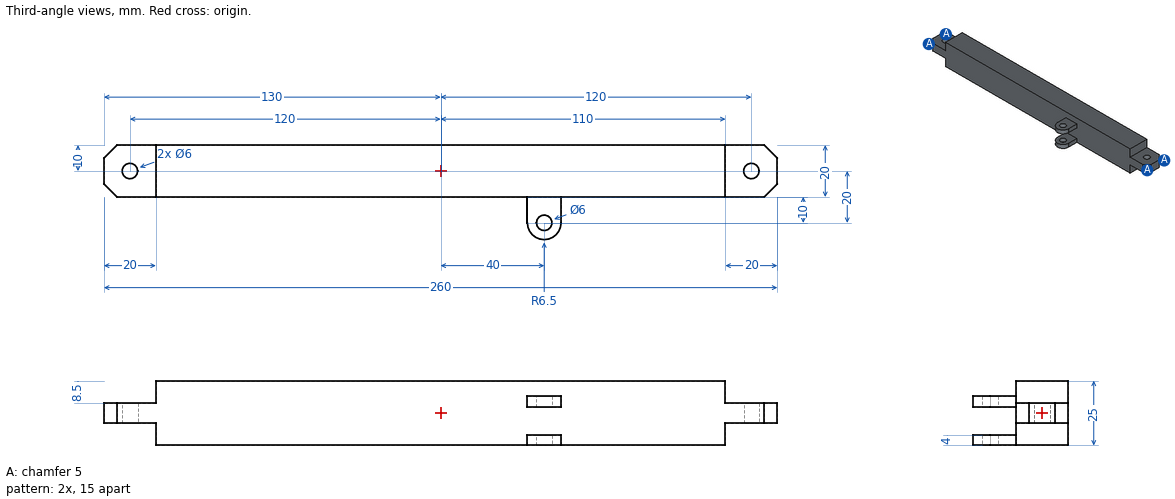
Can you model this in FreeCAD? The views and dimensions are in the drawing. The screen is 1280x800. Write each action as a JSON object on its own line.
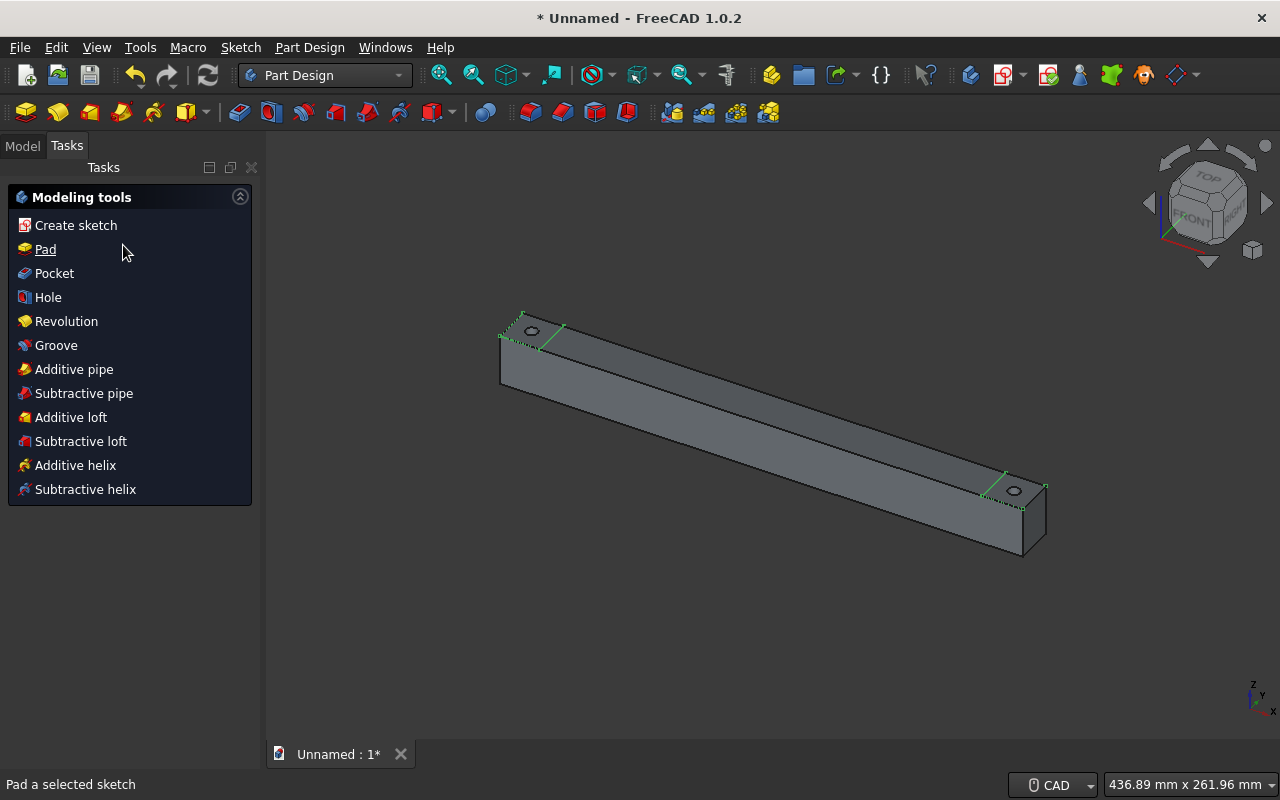
{"action": "left_click", "coordinate": [240, 112]}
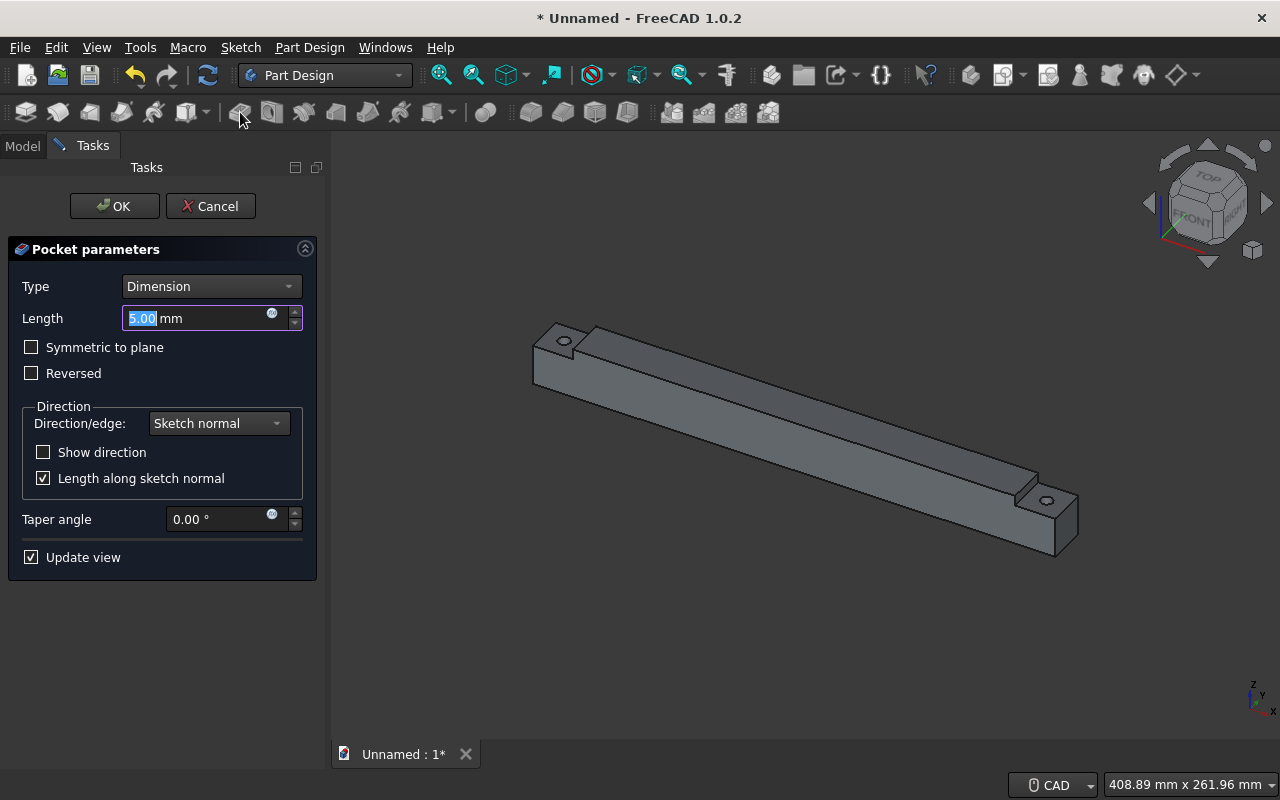
{"action": "type", "text": "8.5"}
{"action": "key", "text": "Tab"}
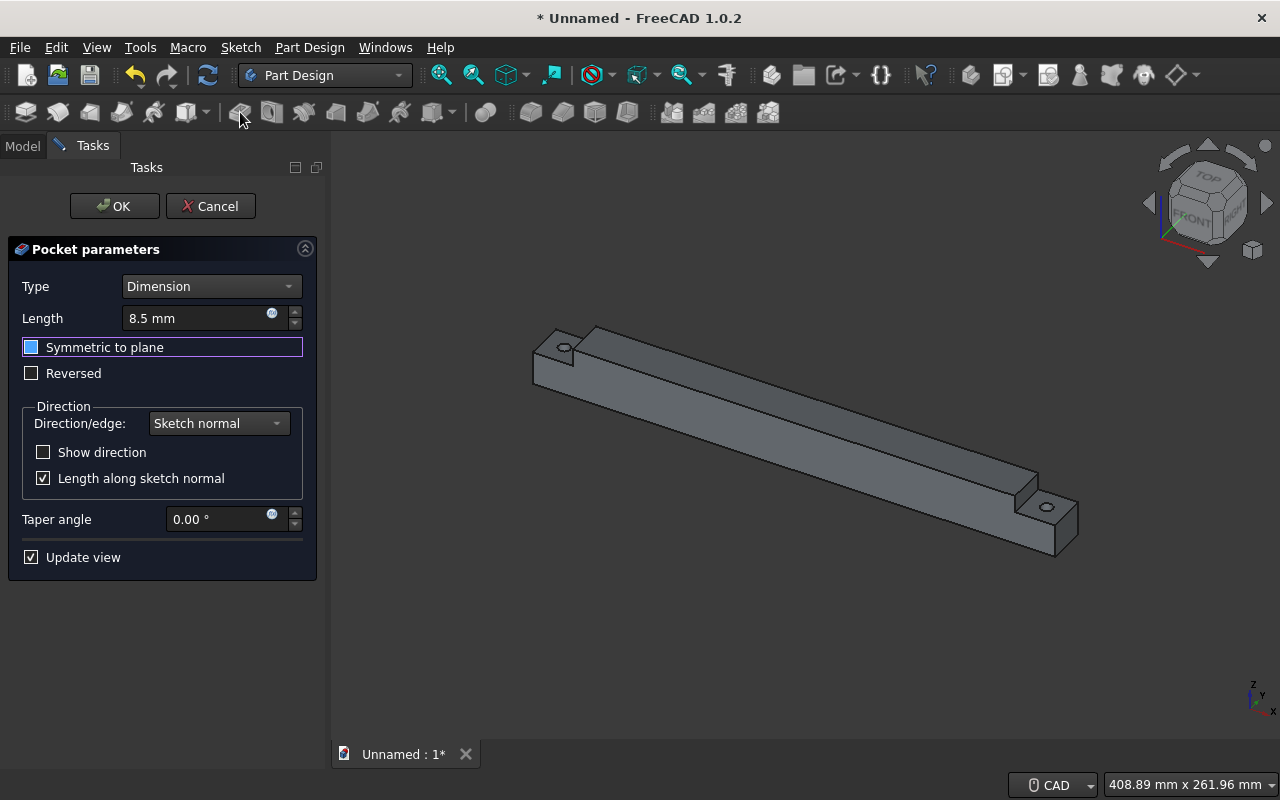
{"action": "left_click", "coordinate": [115, 206]}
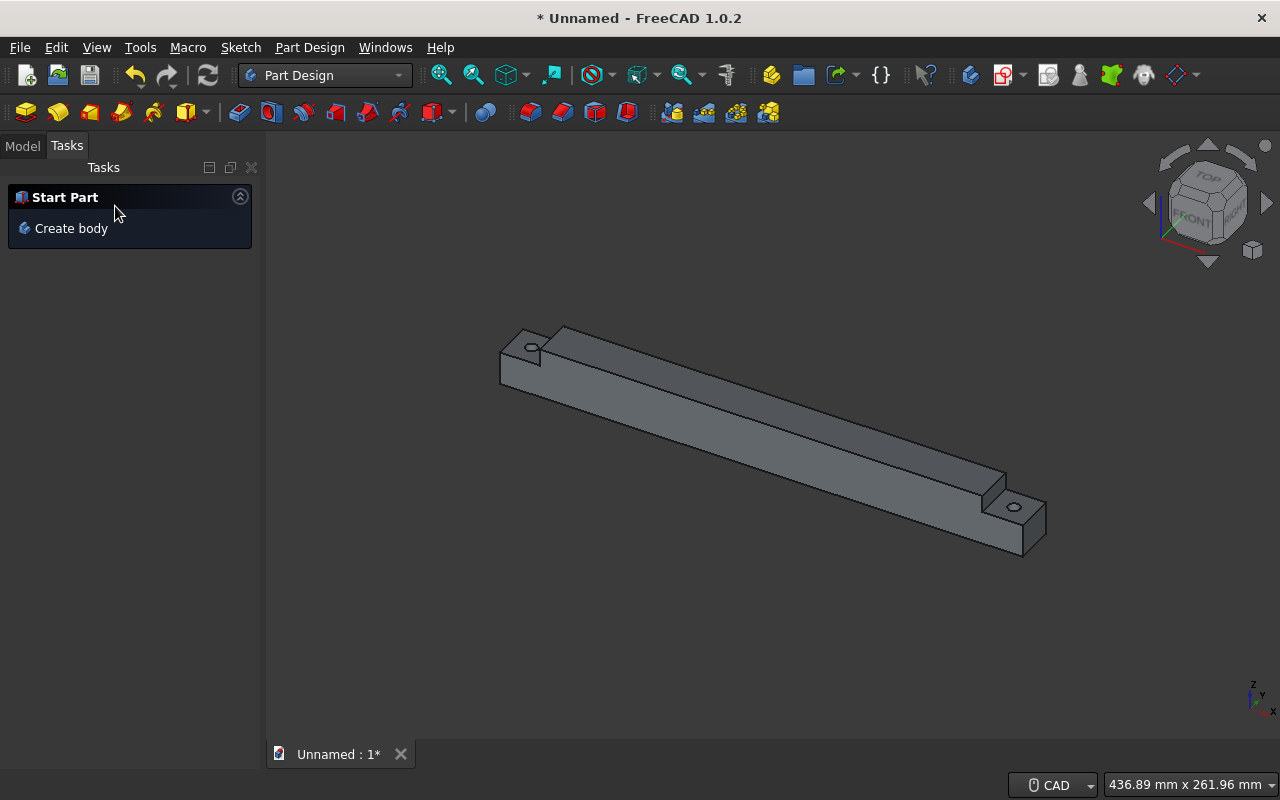
{"action": "left_click", "coordinate": [23, 145]}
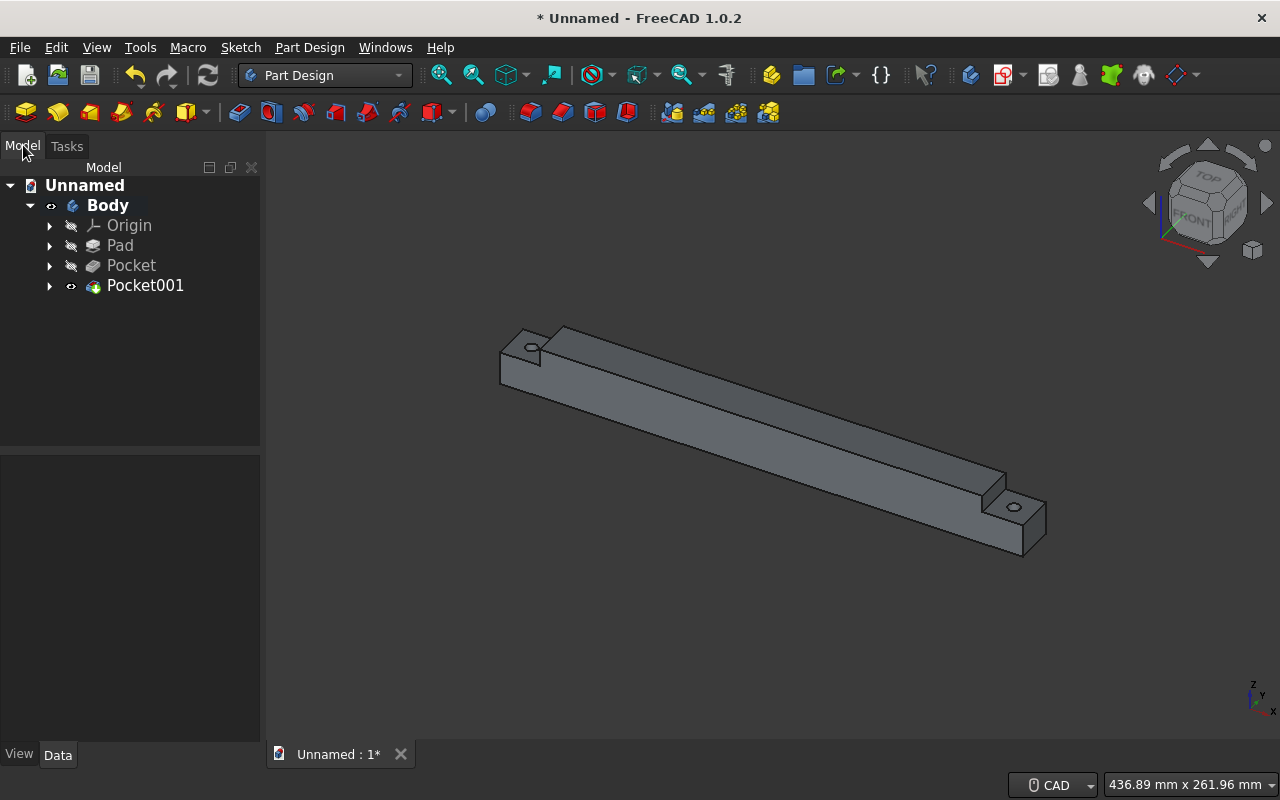
{"action": "left_click", "coordinate": [116, 286]}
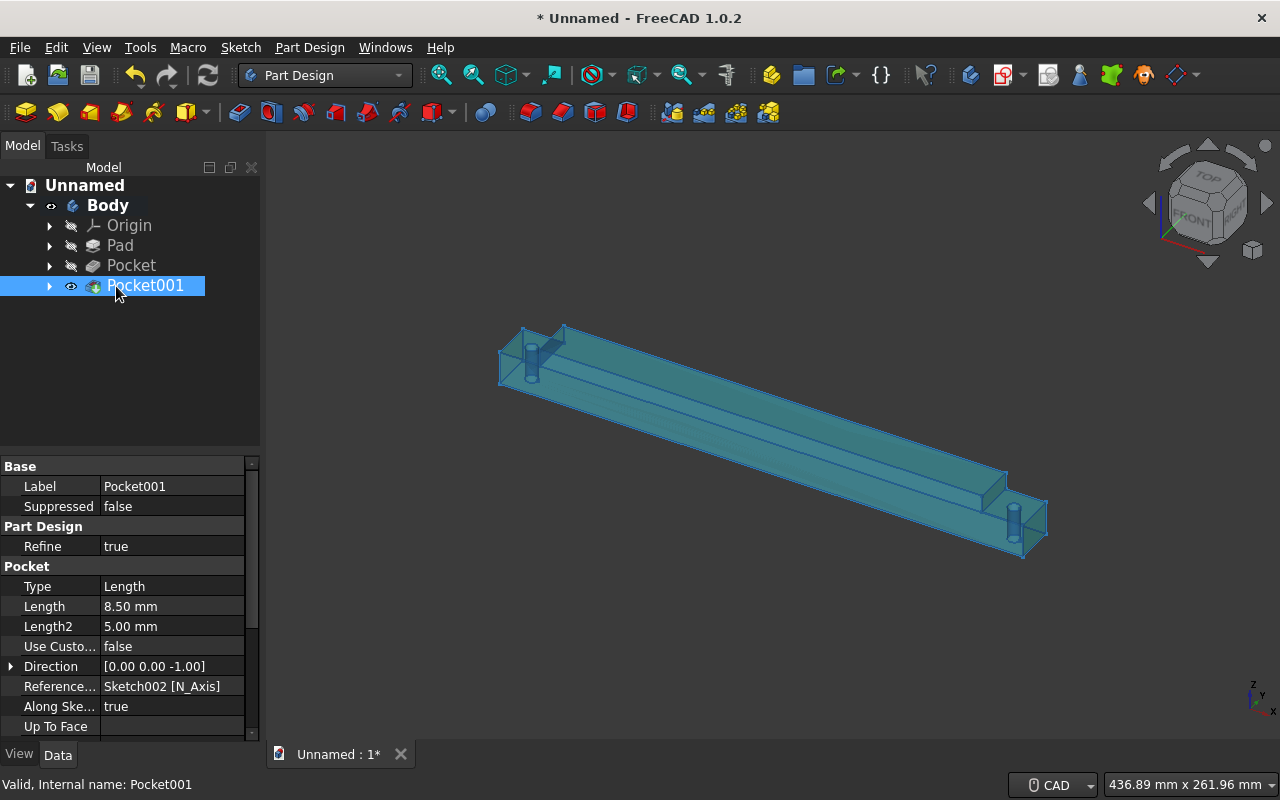
{"action": "left_click", "coordinate": [672, 112]}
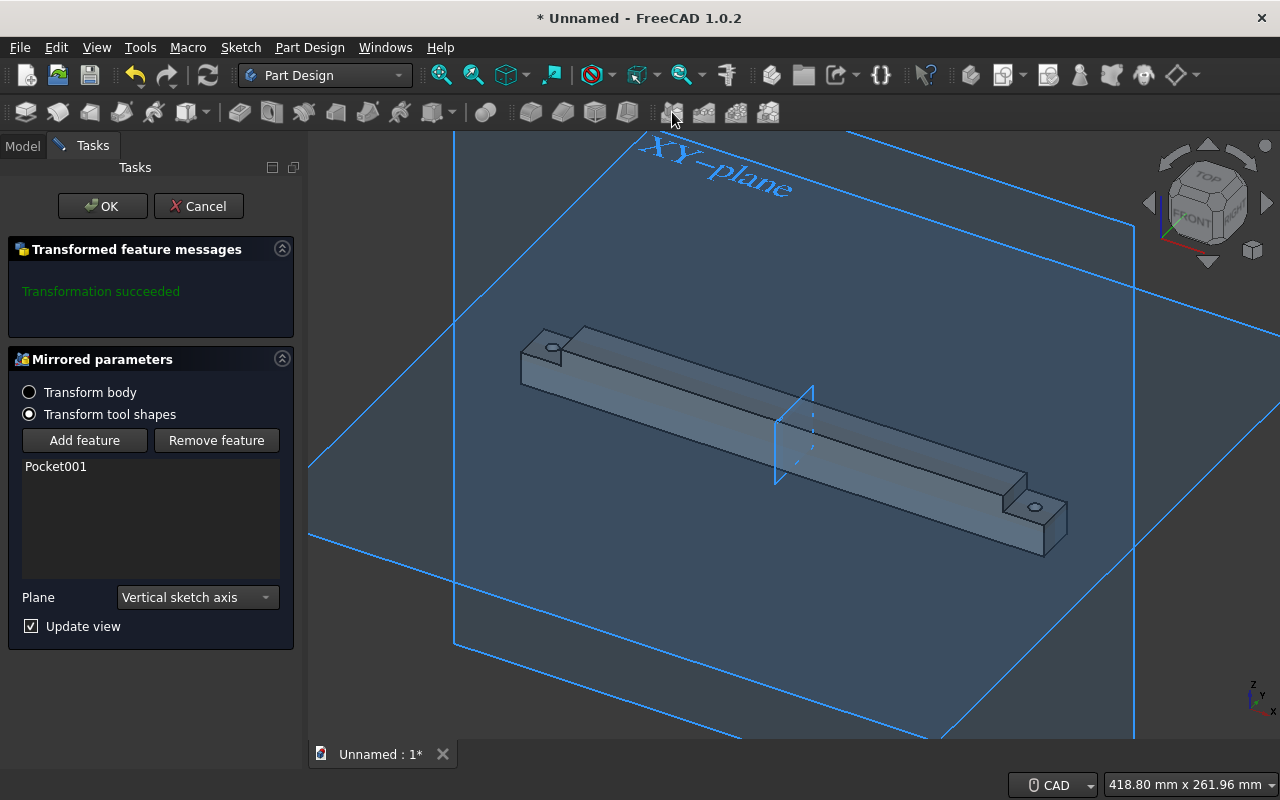
{"action": "left_click", "coordinate": [198, 598]}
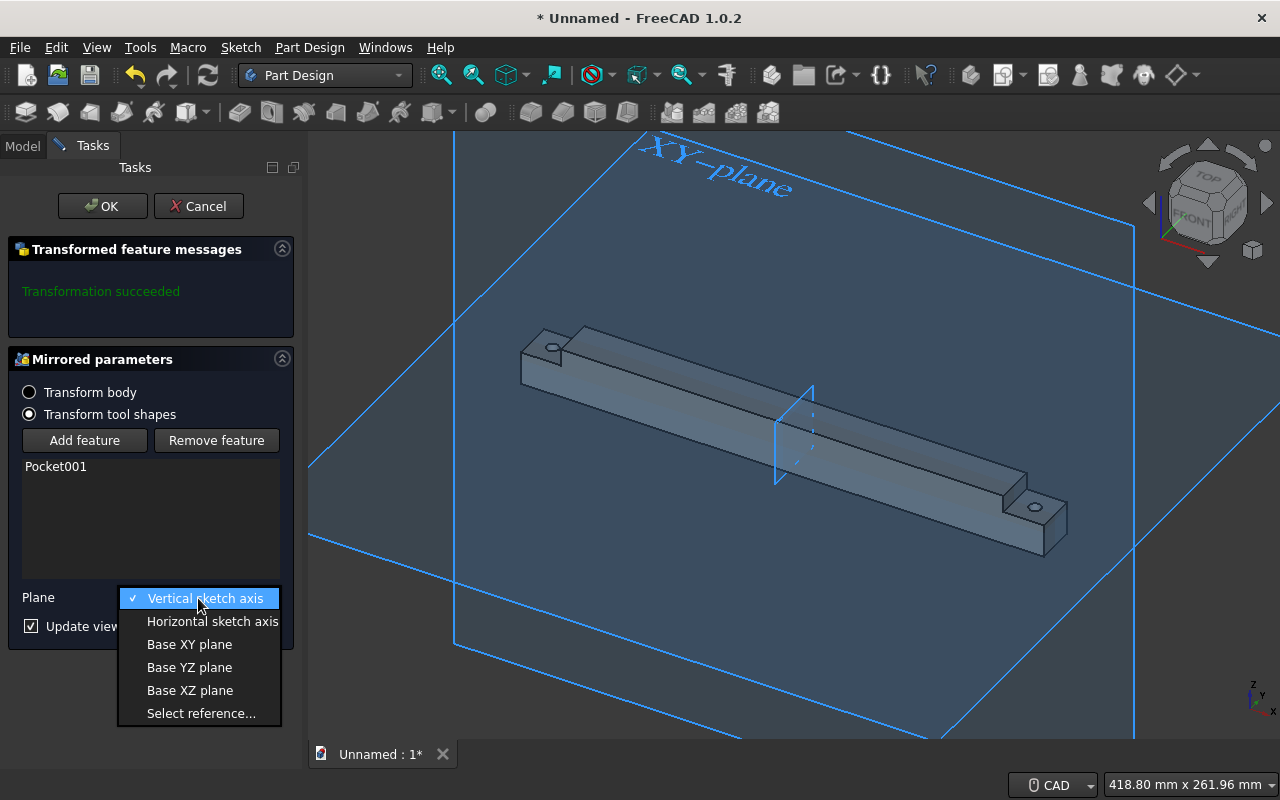
{"action": "left_click", "coordinate": [198, 644]}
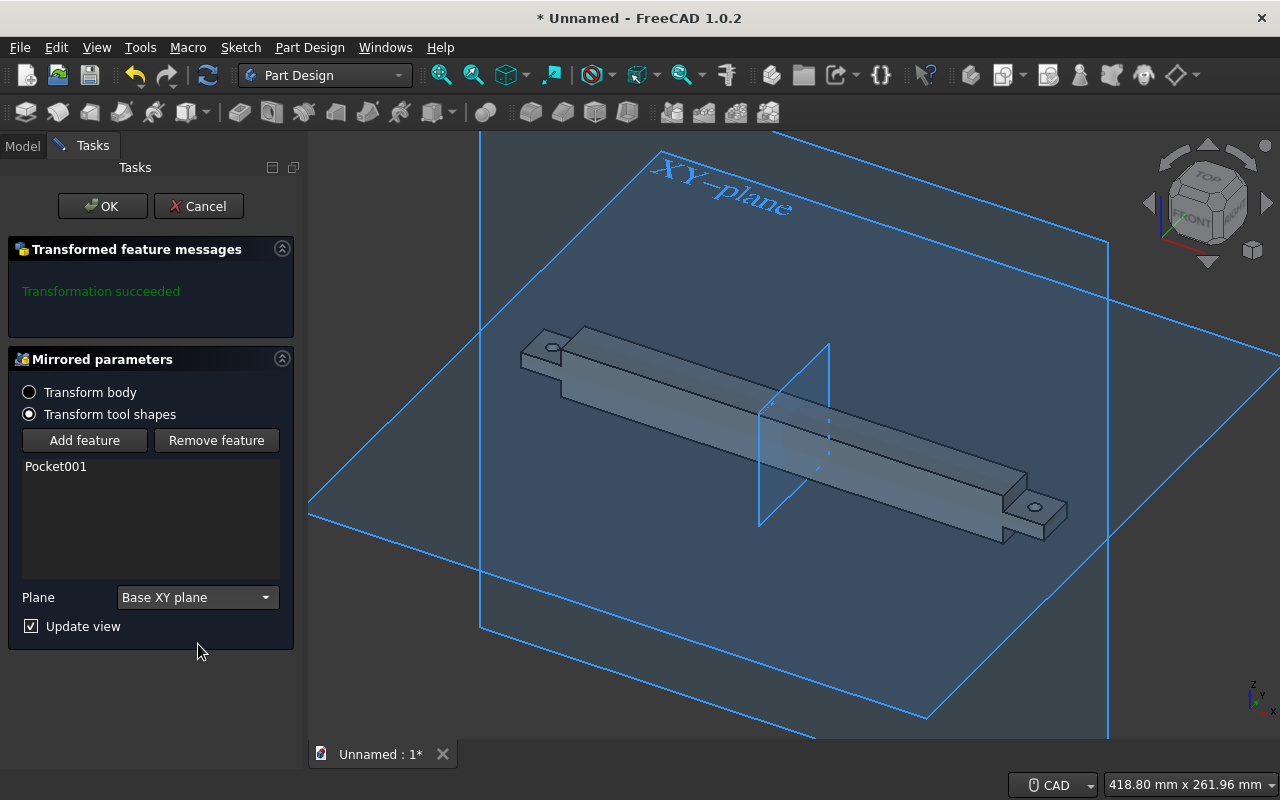
{"action": "left_click", "coordinate": [103, 206]}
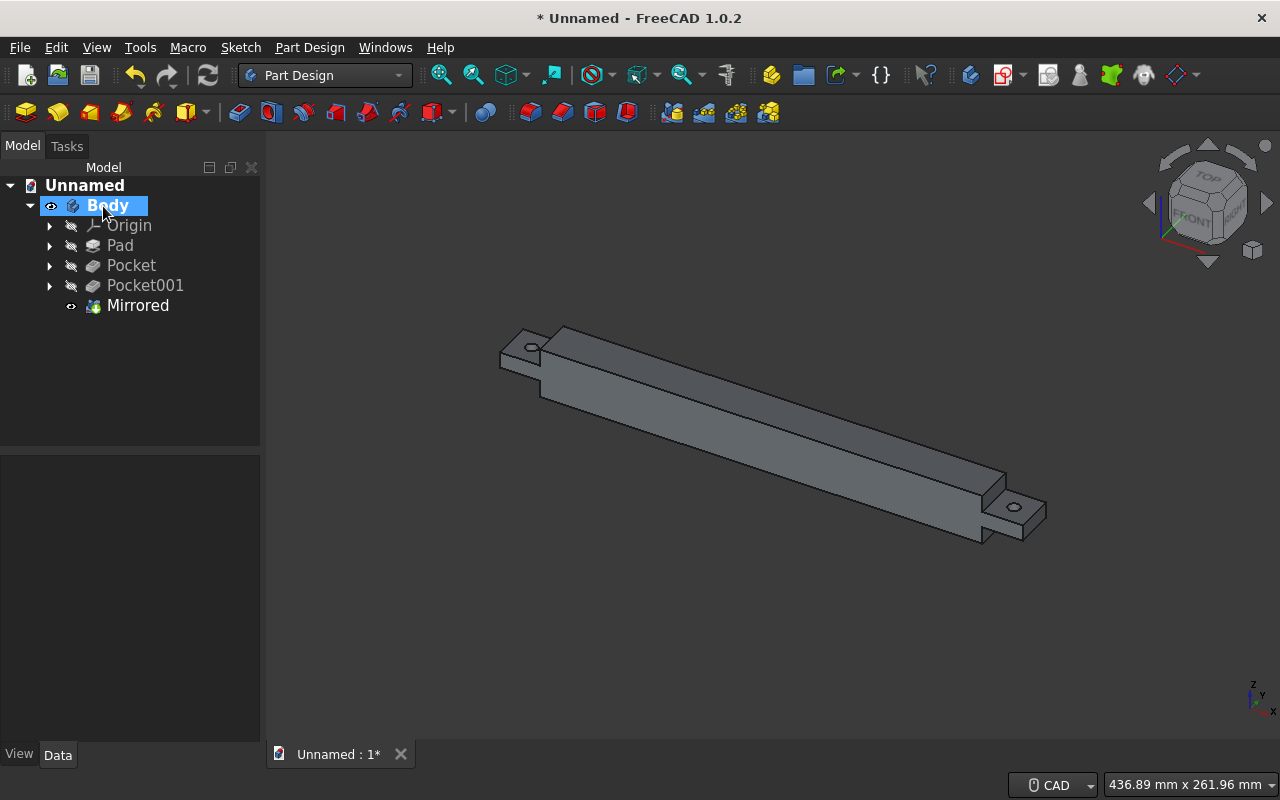
{"action": "left_click", "coordinate": [1023, 532]}